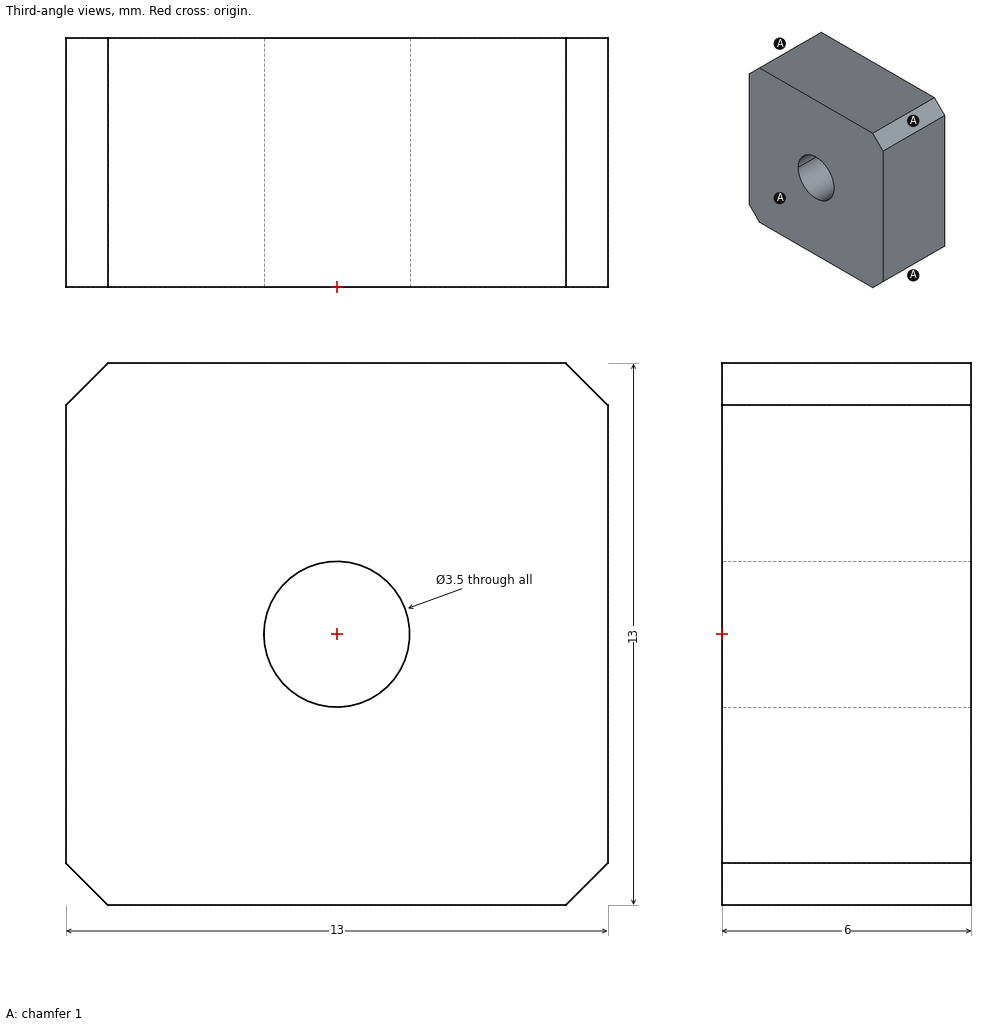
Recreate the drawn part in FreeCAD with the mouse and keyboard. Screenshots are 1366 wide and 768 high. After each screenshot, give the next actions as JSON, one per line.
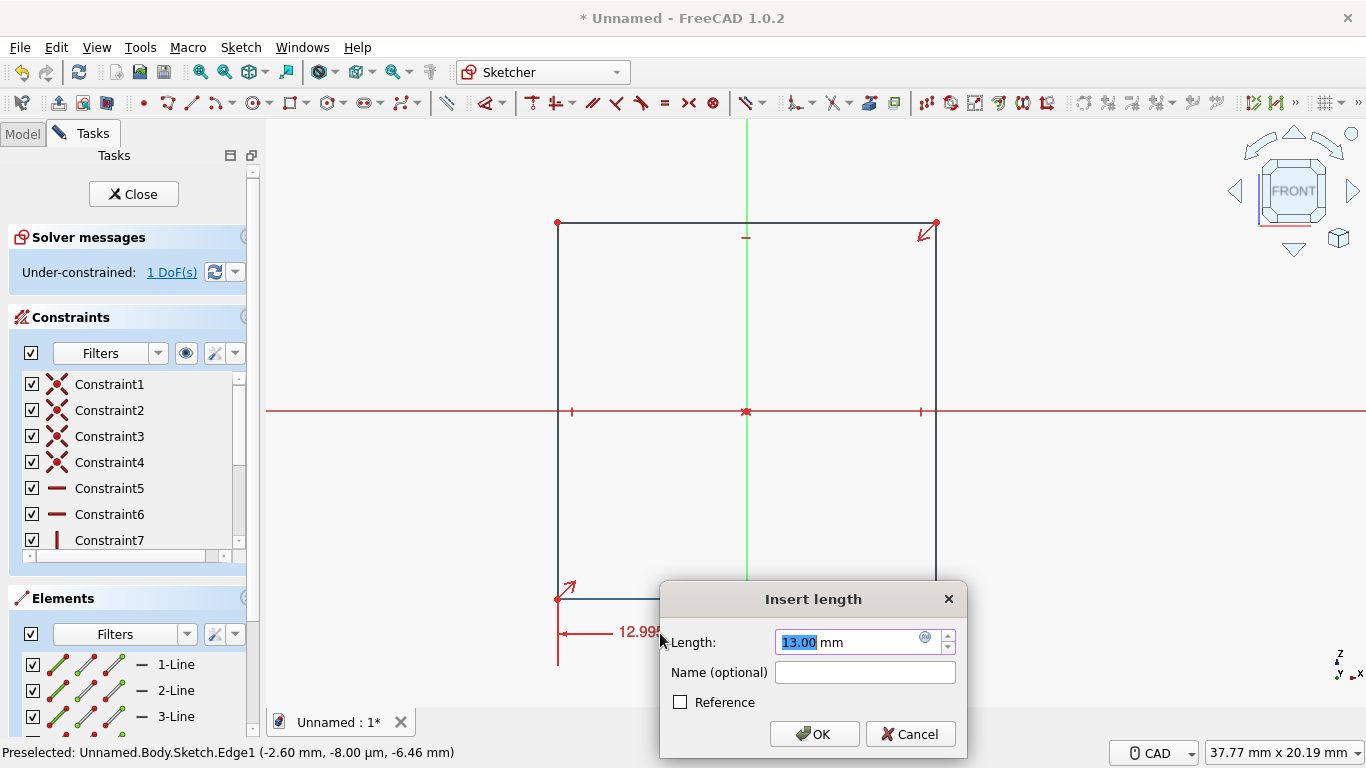
{"action": "type", "text": "13"}
{"action": "key", "text": "Return"}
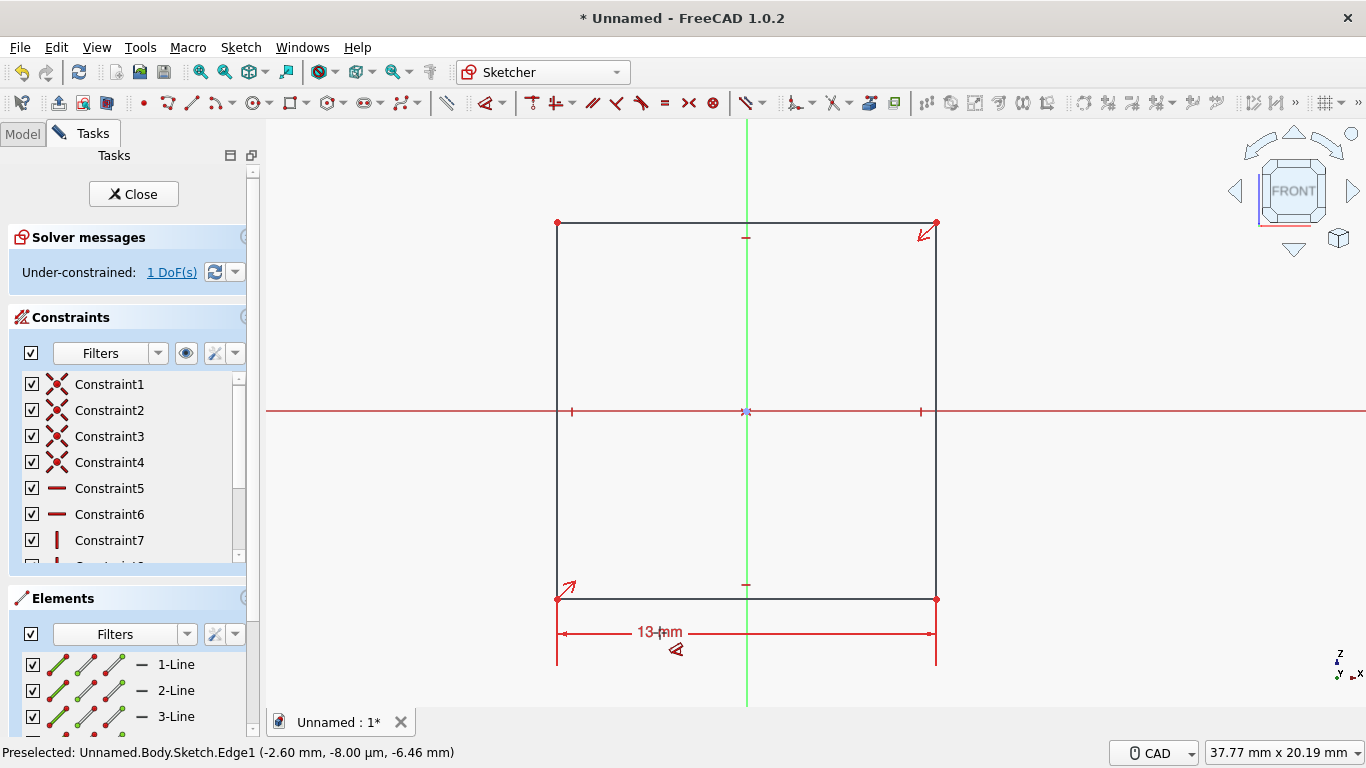
{"action": "left_click", "coordinate": [936, 486]}
{"action": "left_click", "coordinate": [970, 325]}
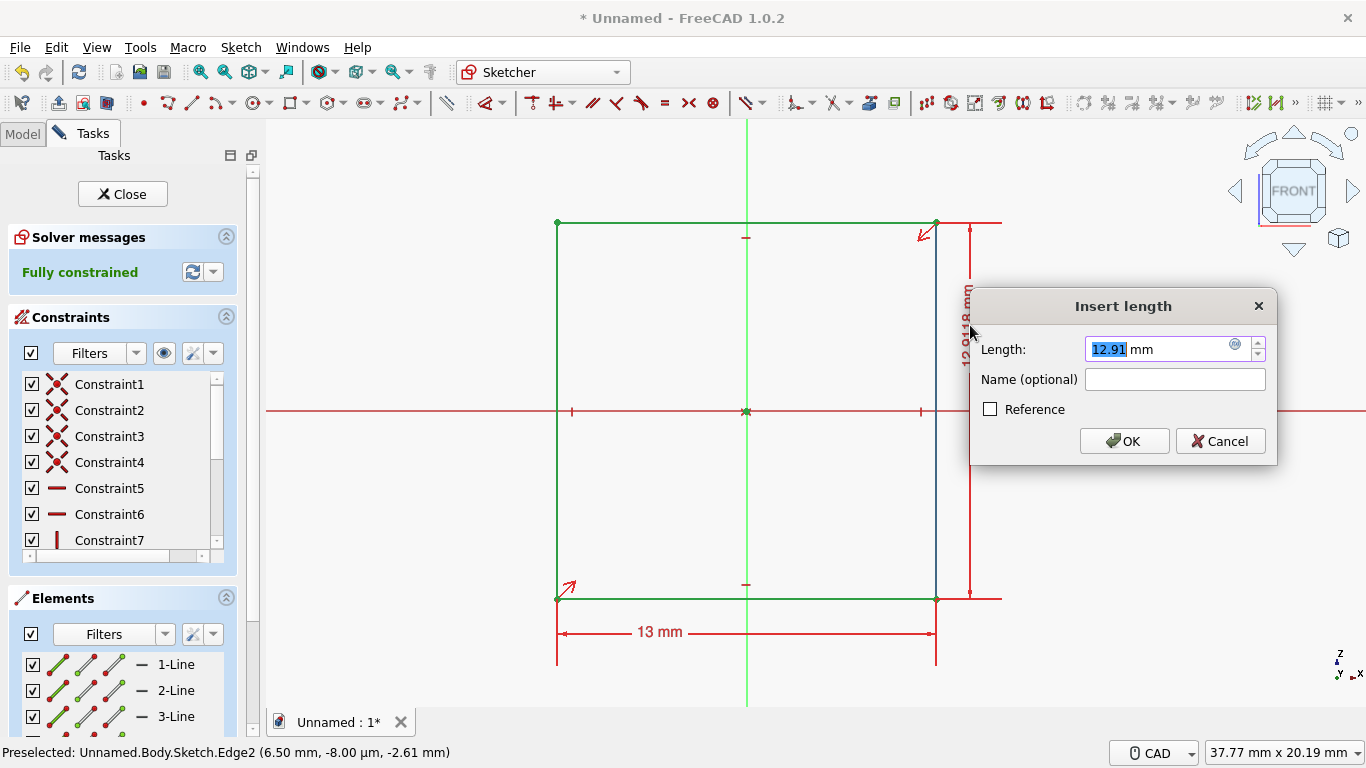
{"action": "type", "text": "13"}
{"action": "key", "text": "Return"}
{"action": "key", "text": "Escape"}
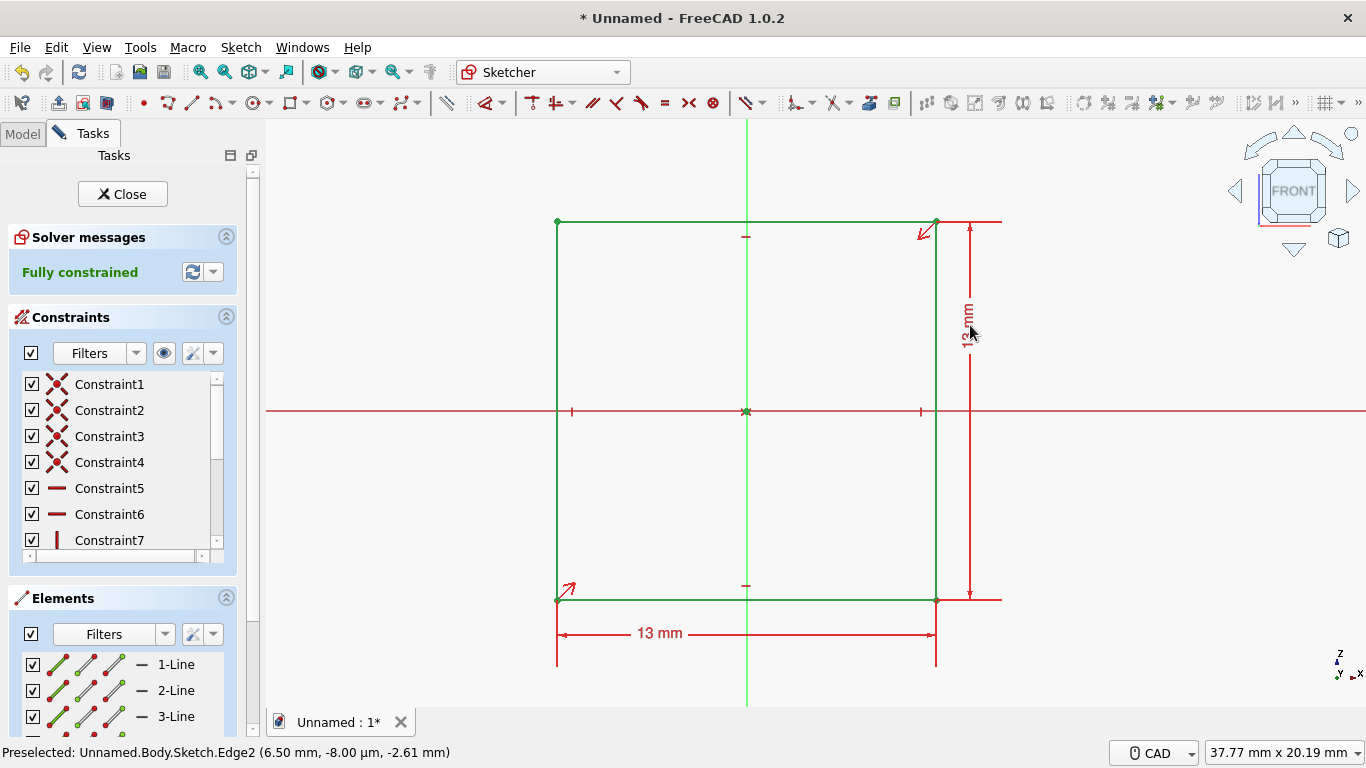
{"action": "left_click", "coordinate": [123, 194]}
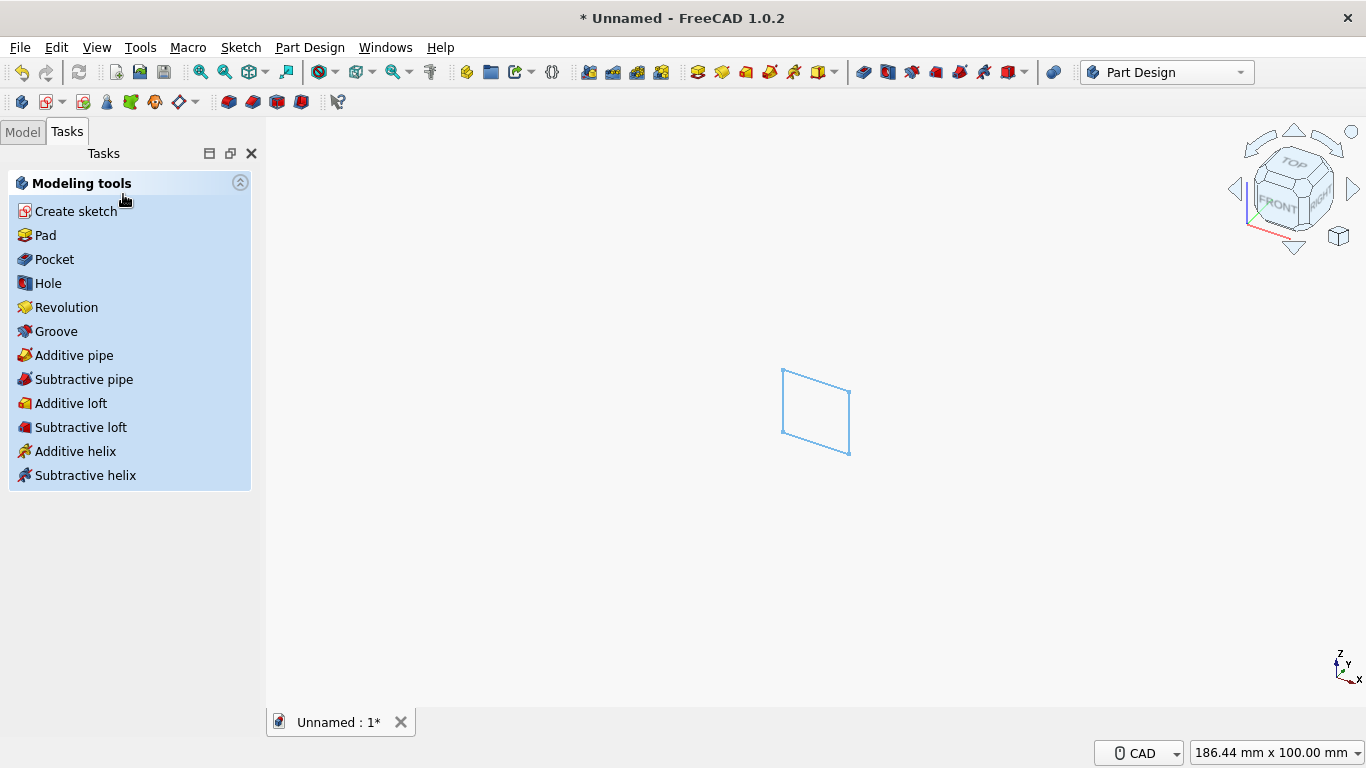
{"action": "left_click", "coordinate": [698, 72]}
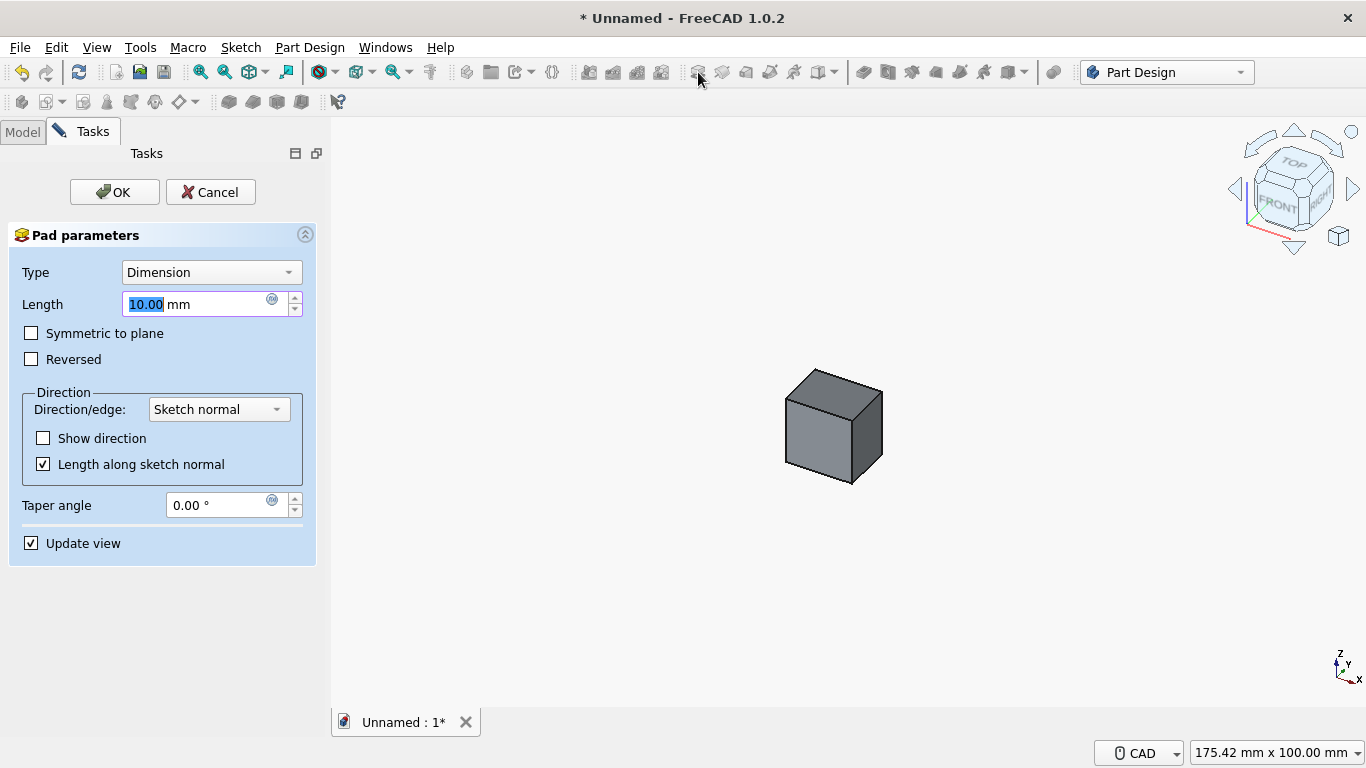
{"action": "type", "text": "6"}
{"action": "key", "text": "Tab"}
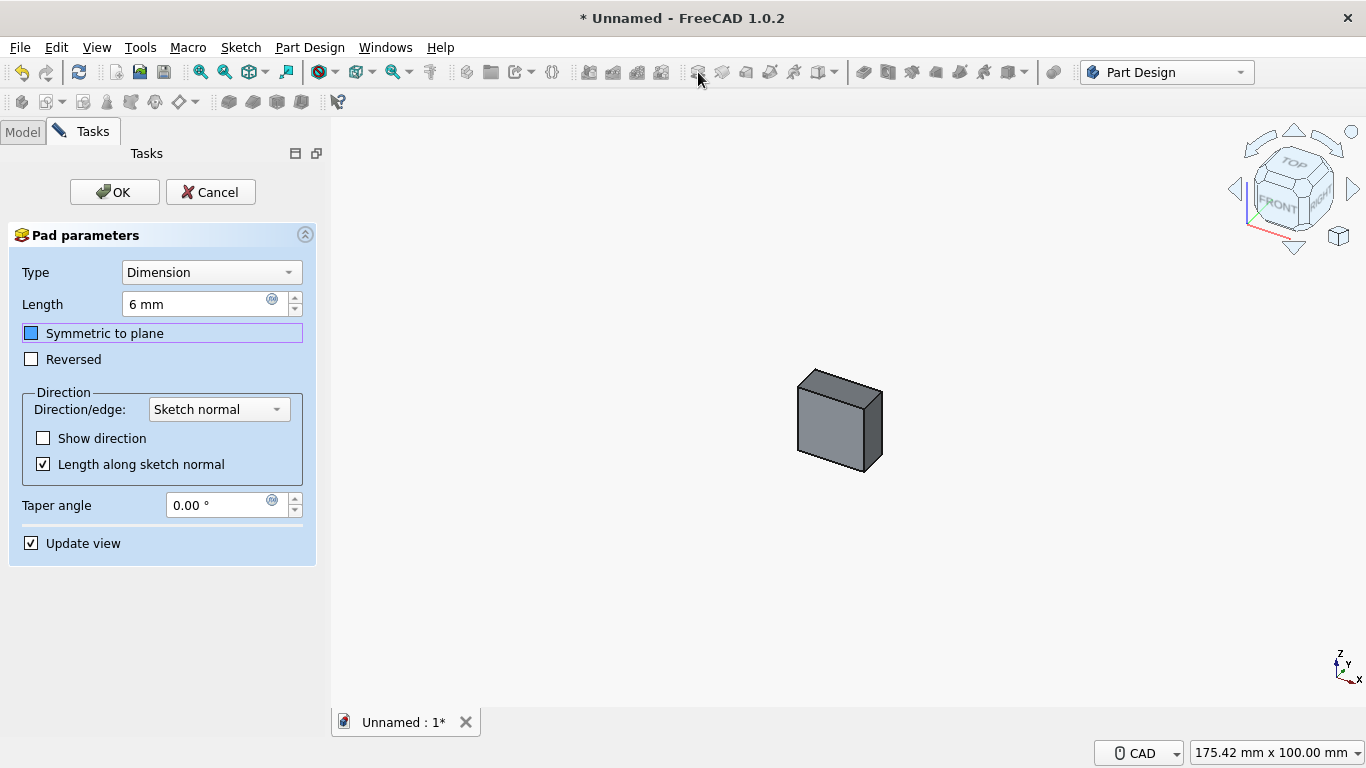
{"action": "left_click", "coordinate": [30, 359]}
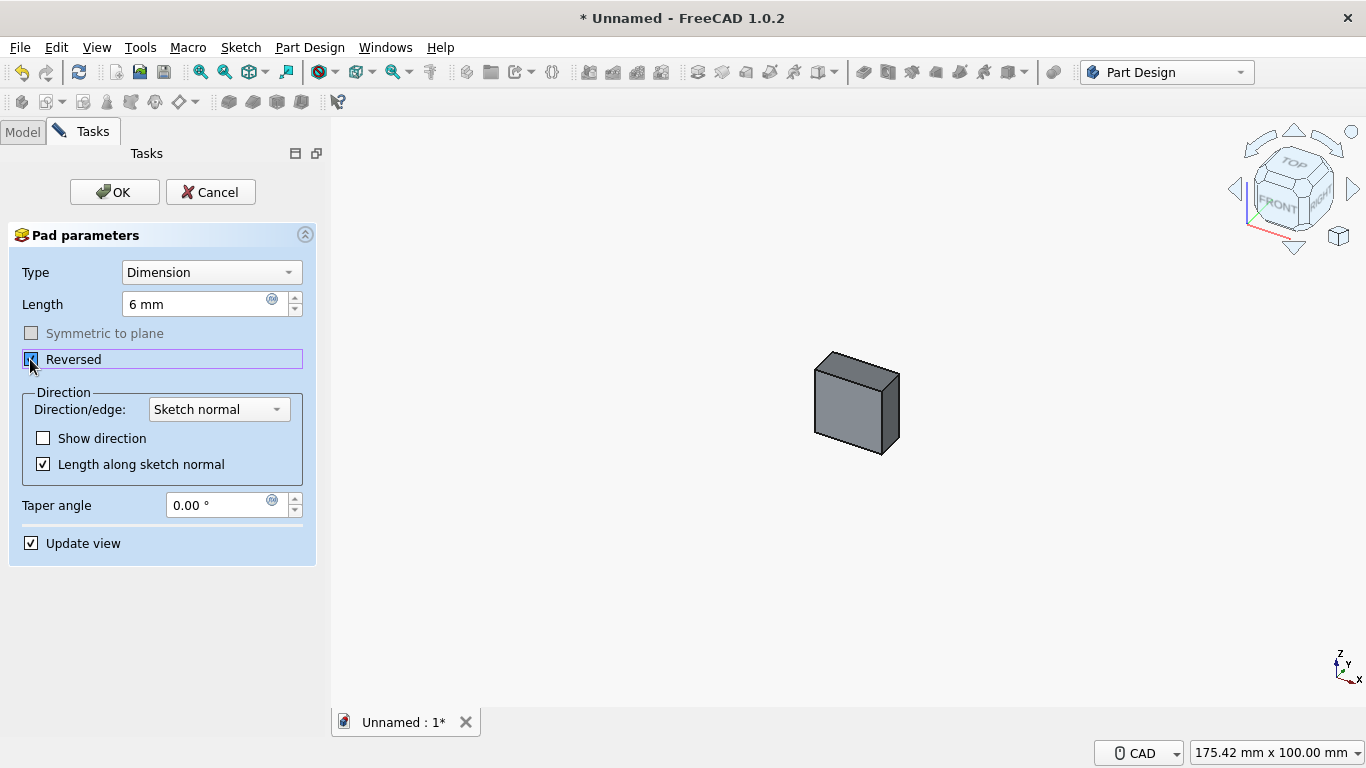
{"action": "left_click", "coordinate": [115, 192]}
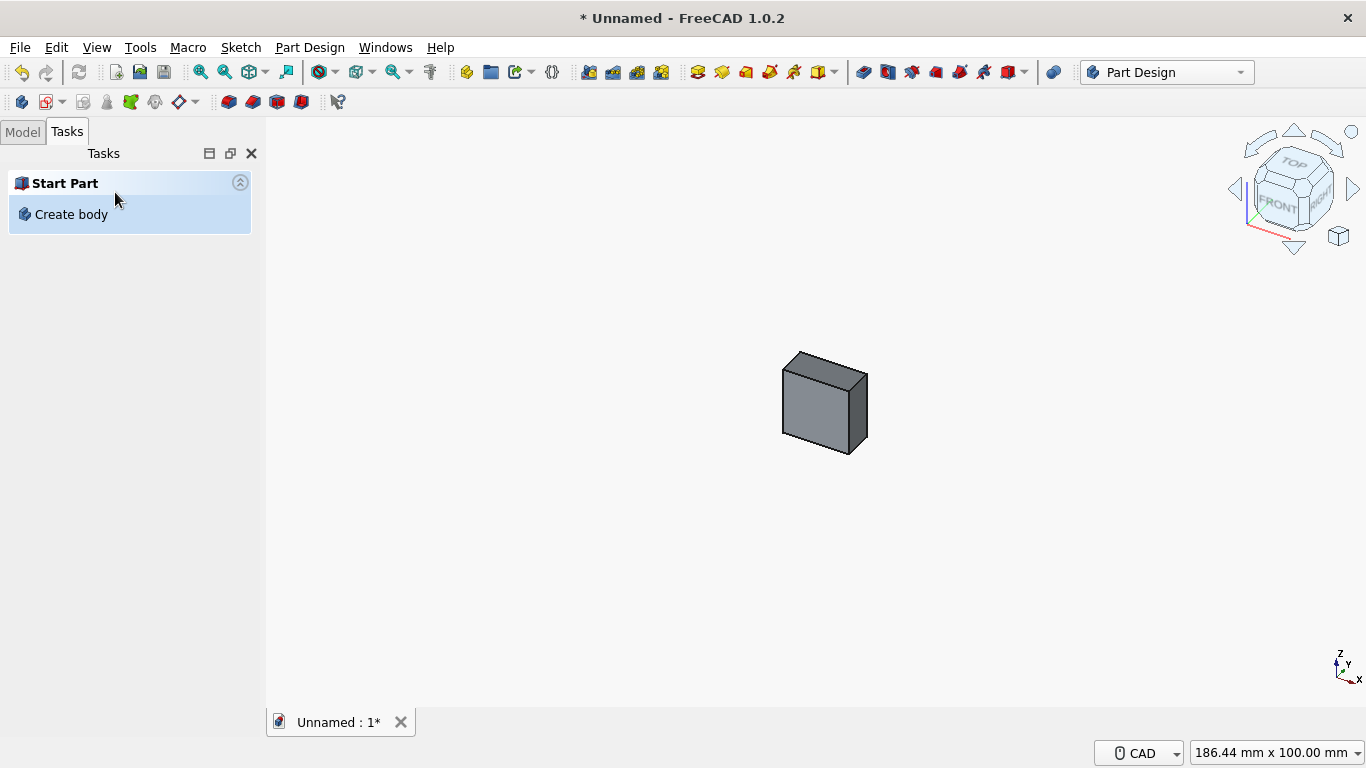
{"action": "left_click", "coordinate": [202, 72]}